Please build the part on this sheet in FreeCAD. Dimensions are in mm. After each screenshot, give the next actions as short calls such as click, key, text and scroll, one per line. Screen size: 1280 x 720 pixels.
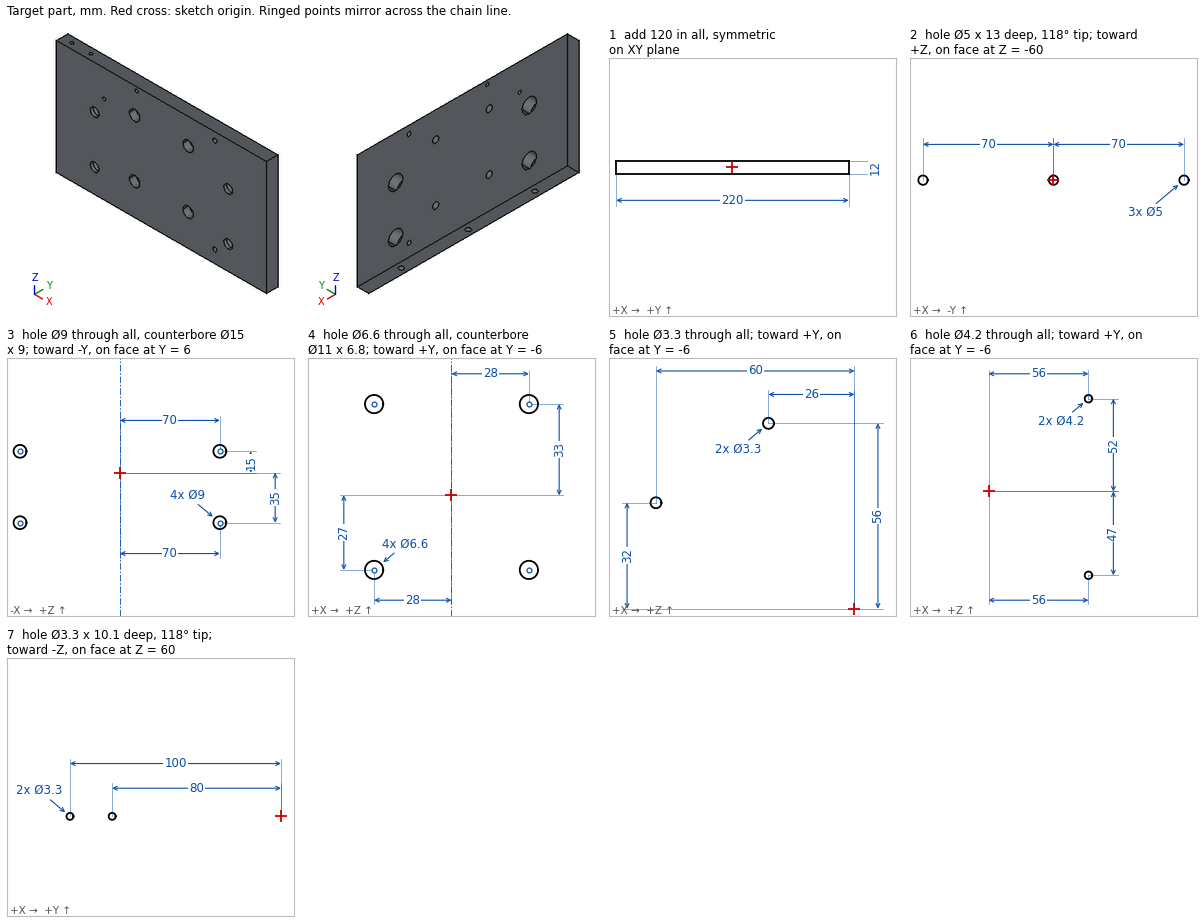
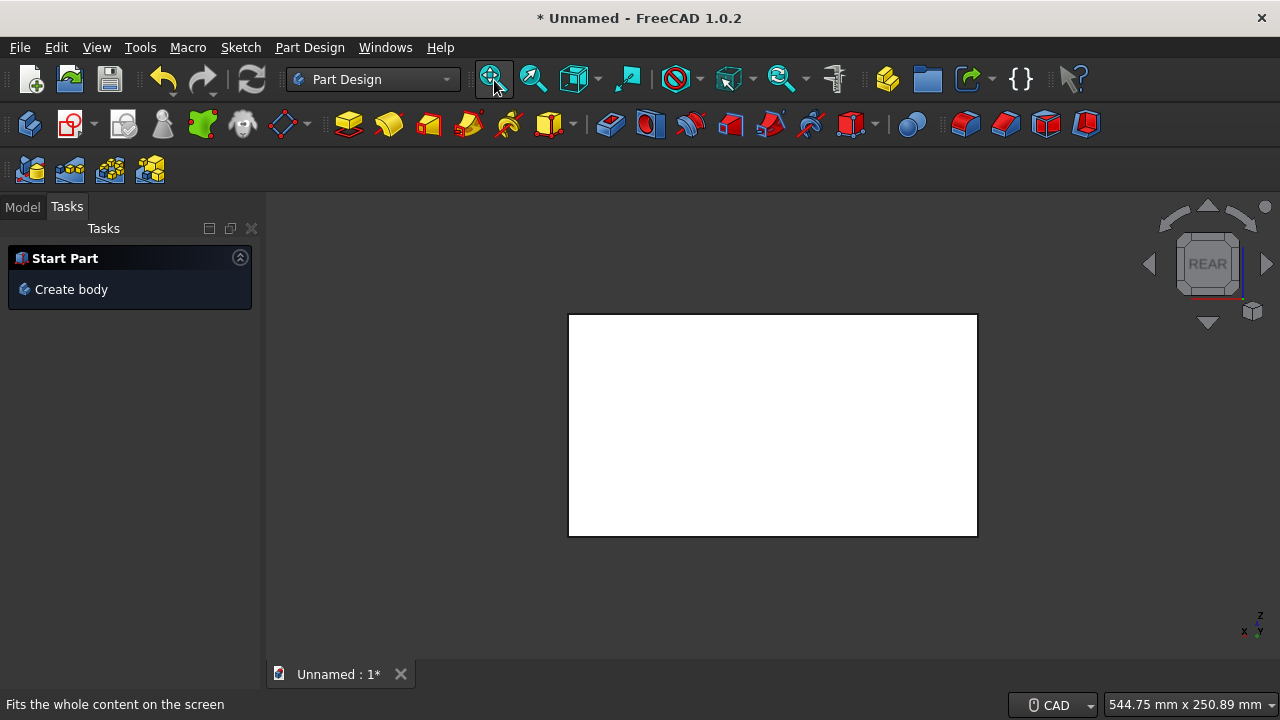
click(714, 425)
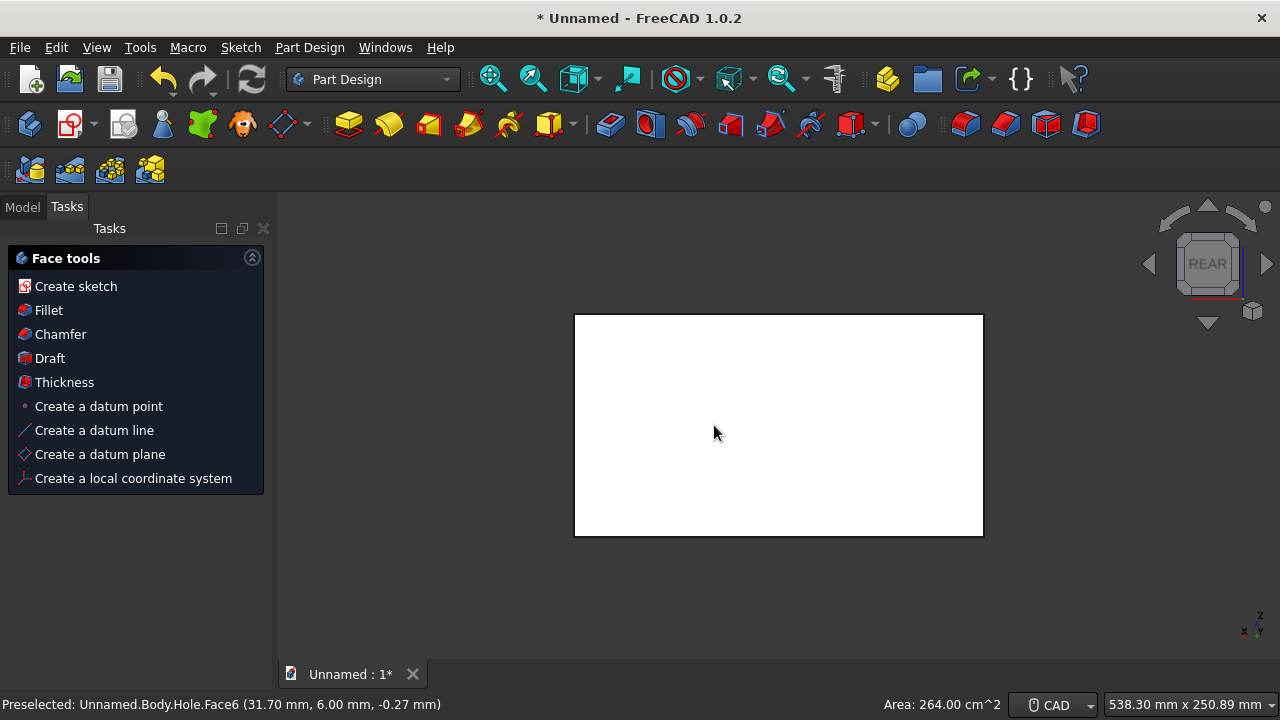
click(70, 124)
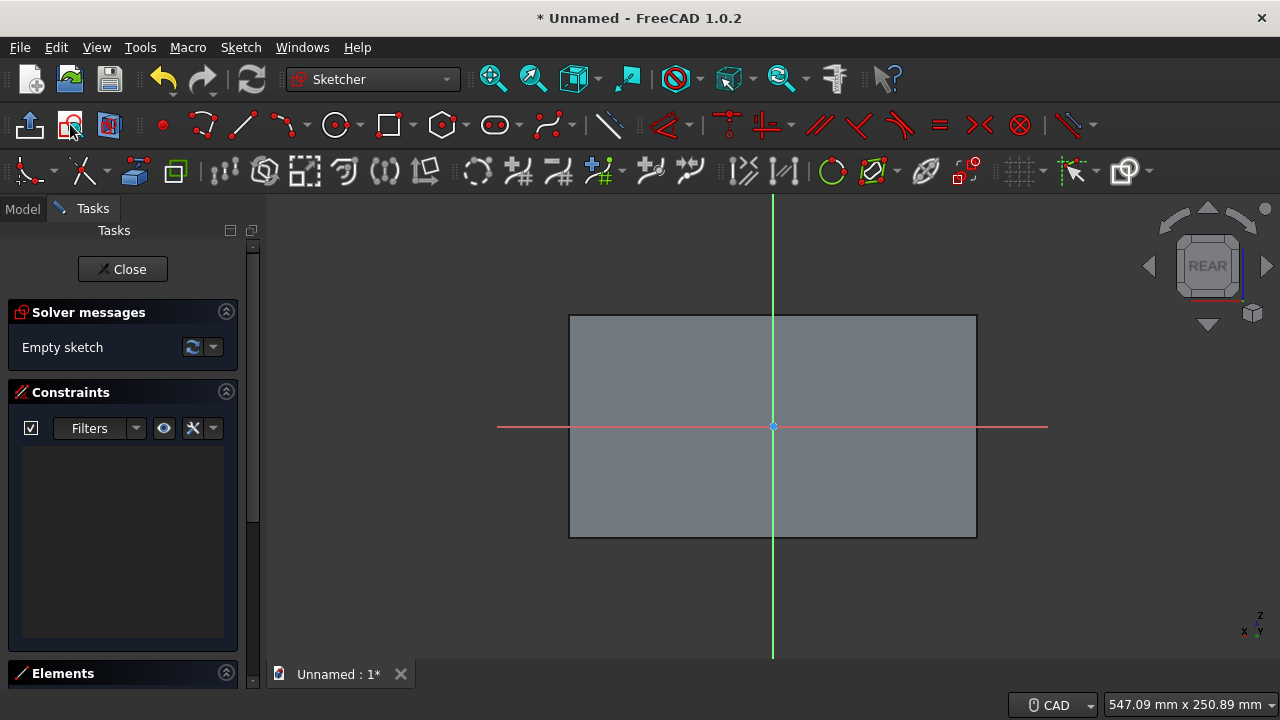
scroll(829, 460, up, 4)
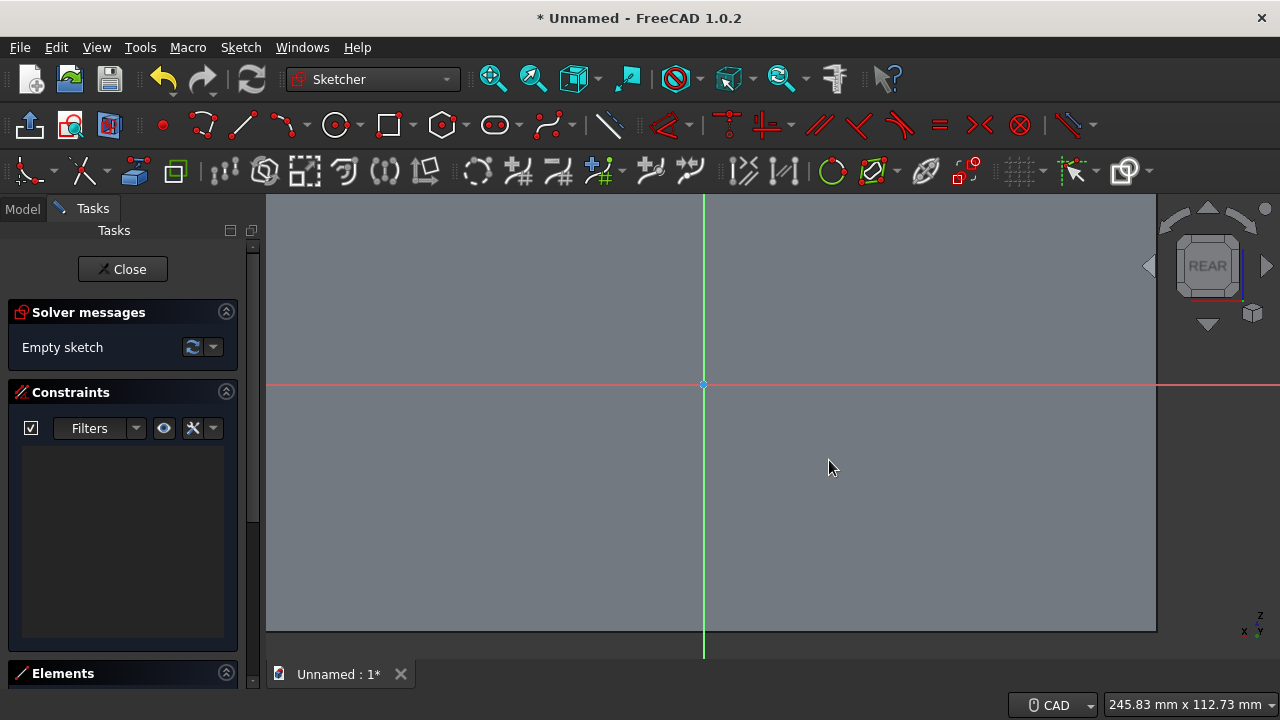
click(336, 126)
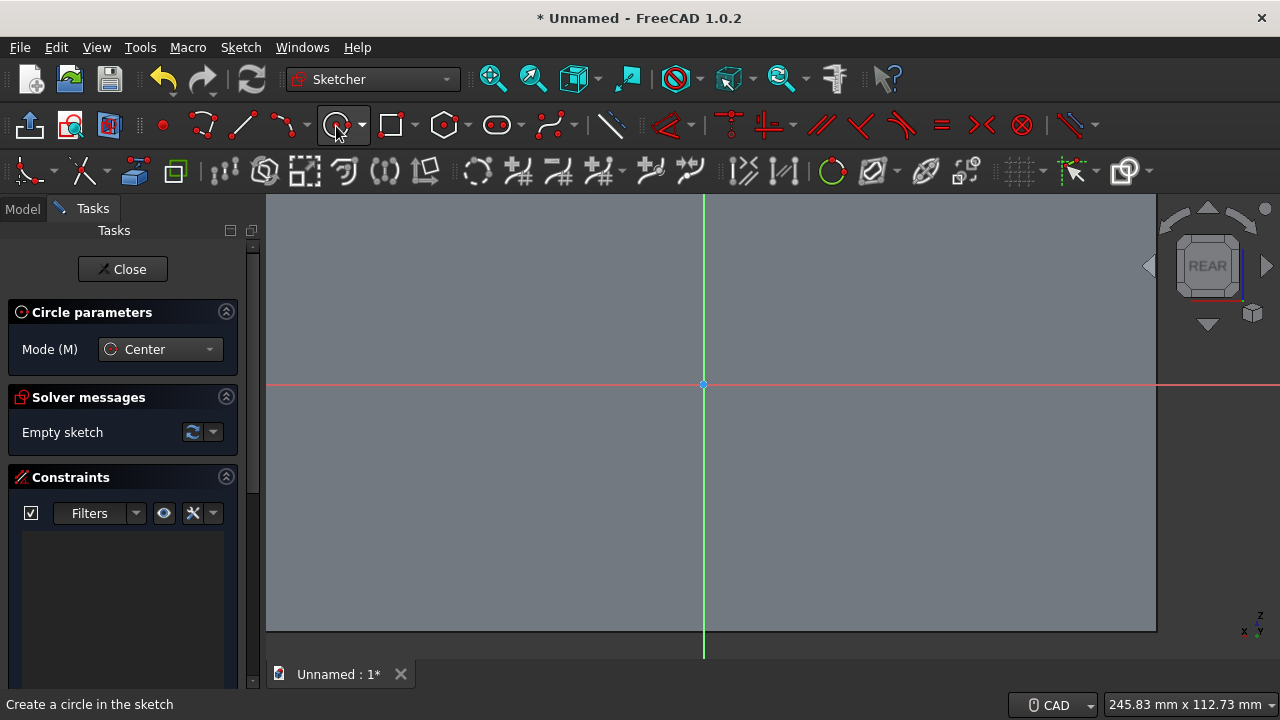
scroll(992, 529, up, 2)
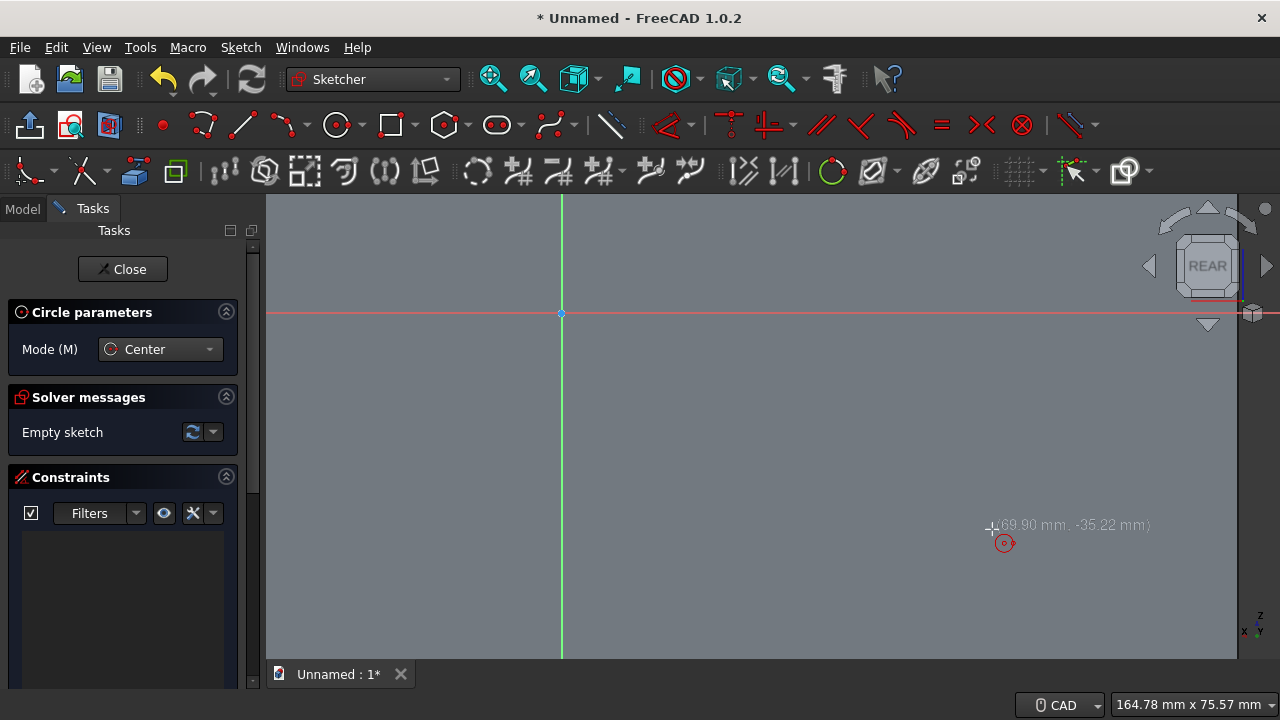
click(992, 529)
move(1012, 509)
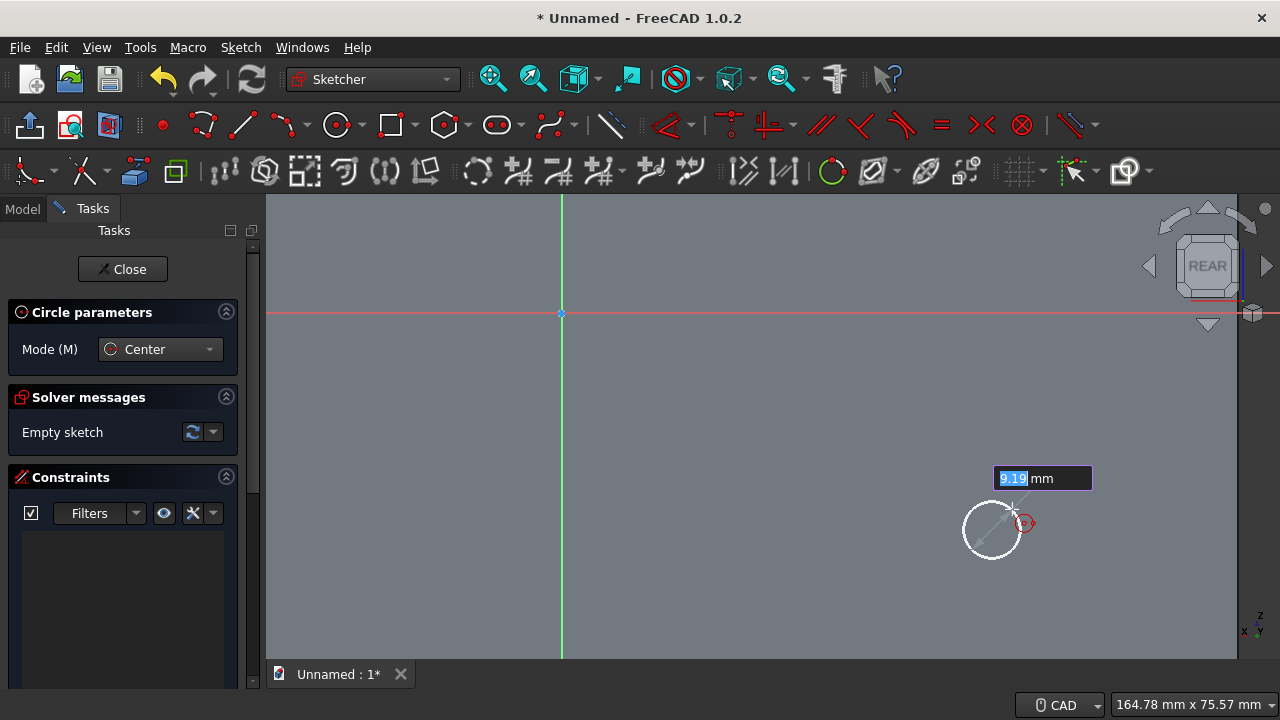
text(9)
key(Return)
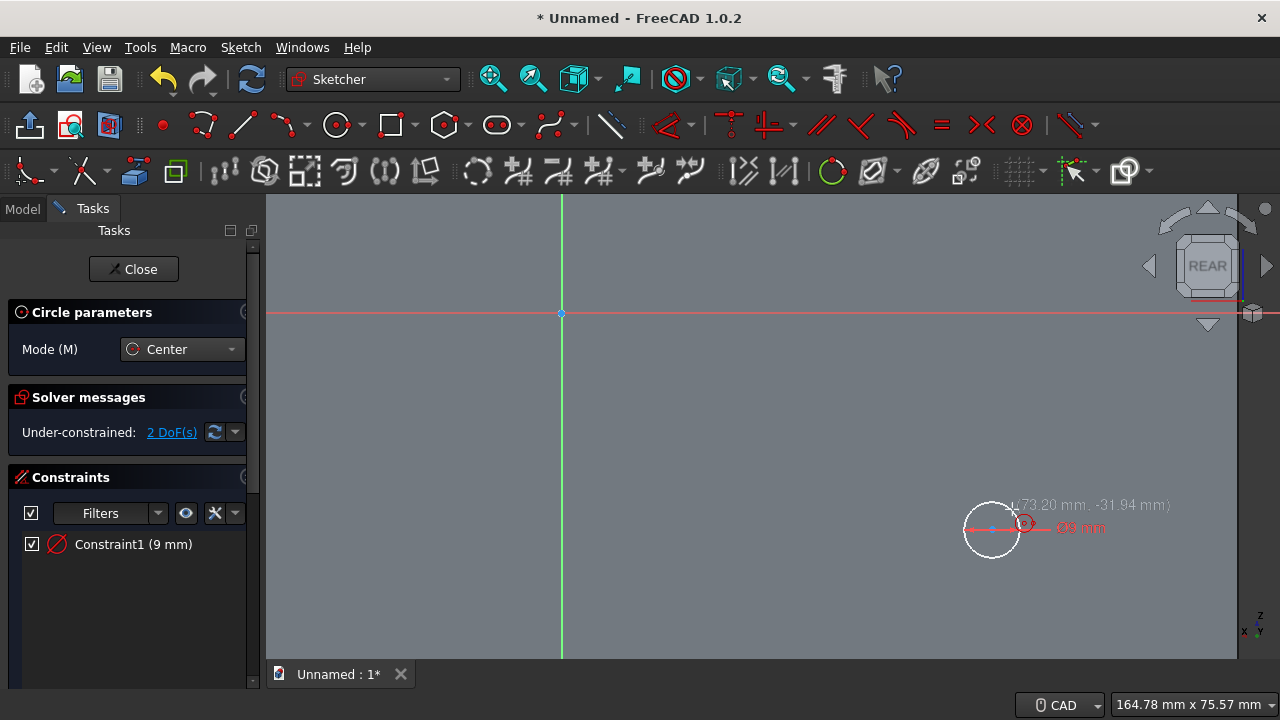
scroll(995, 531, down, 2)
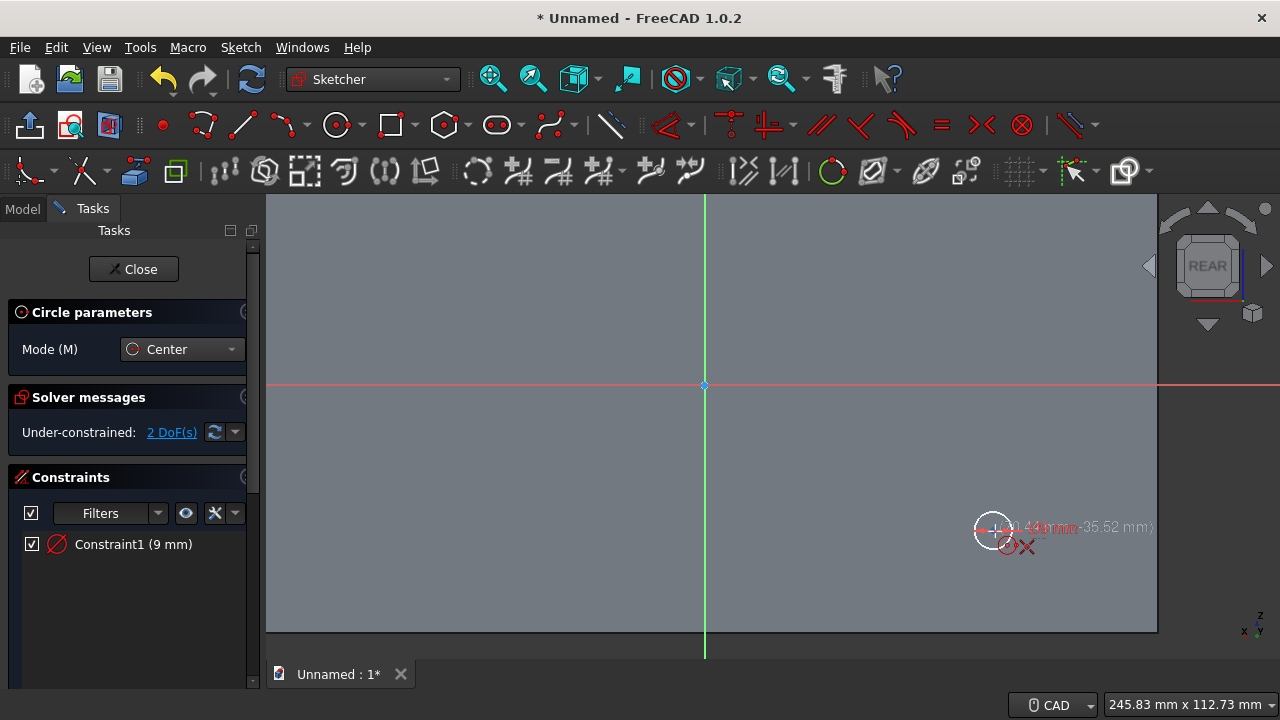
scroll(993, 324, up, 2)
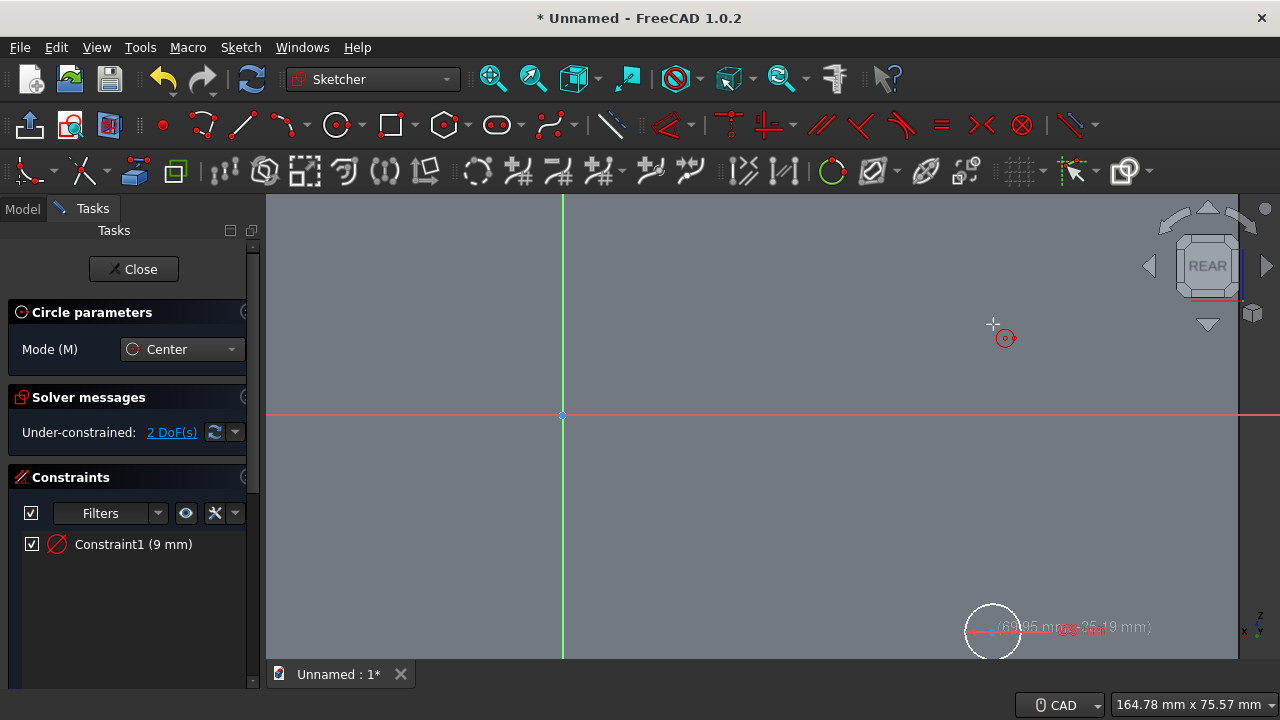
click(993, 323)
move(1013, 304)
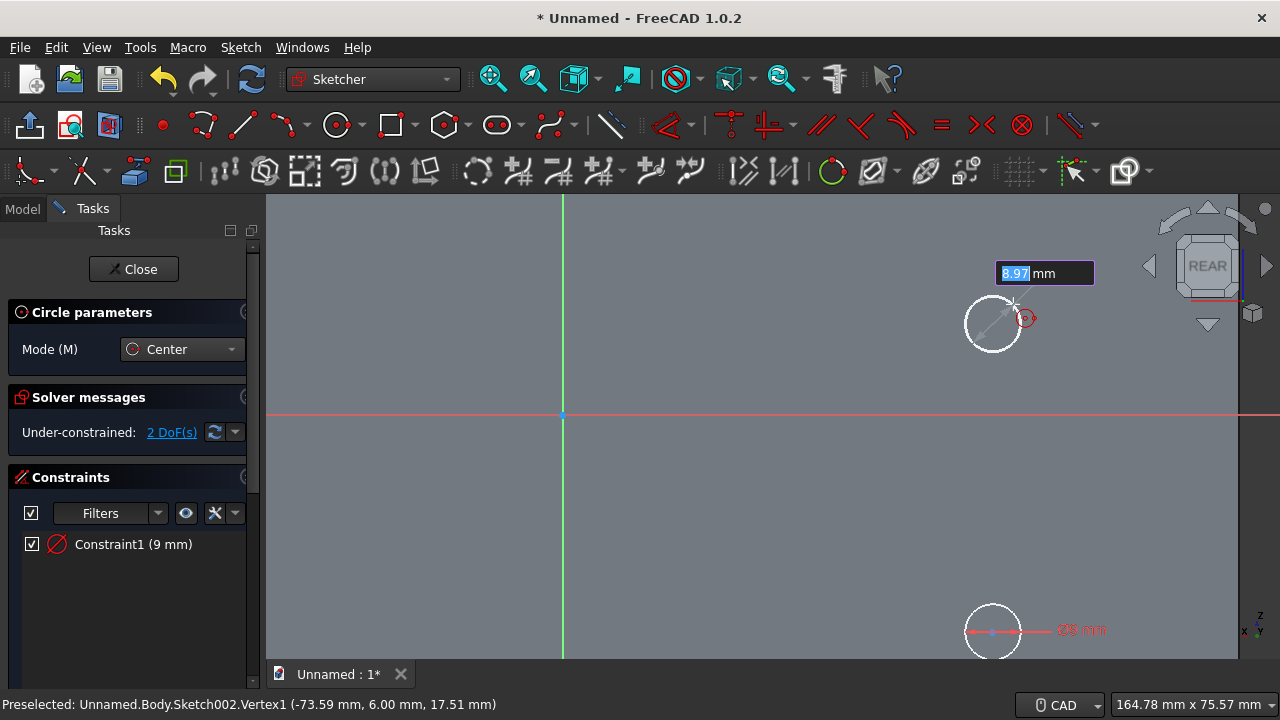
text(9)
key(Return)